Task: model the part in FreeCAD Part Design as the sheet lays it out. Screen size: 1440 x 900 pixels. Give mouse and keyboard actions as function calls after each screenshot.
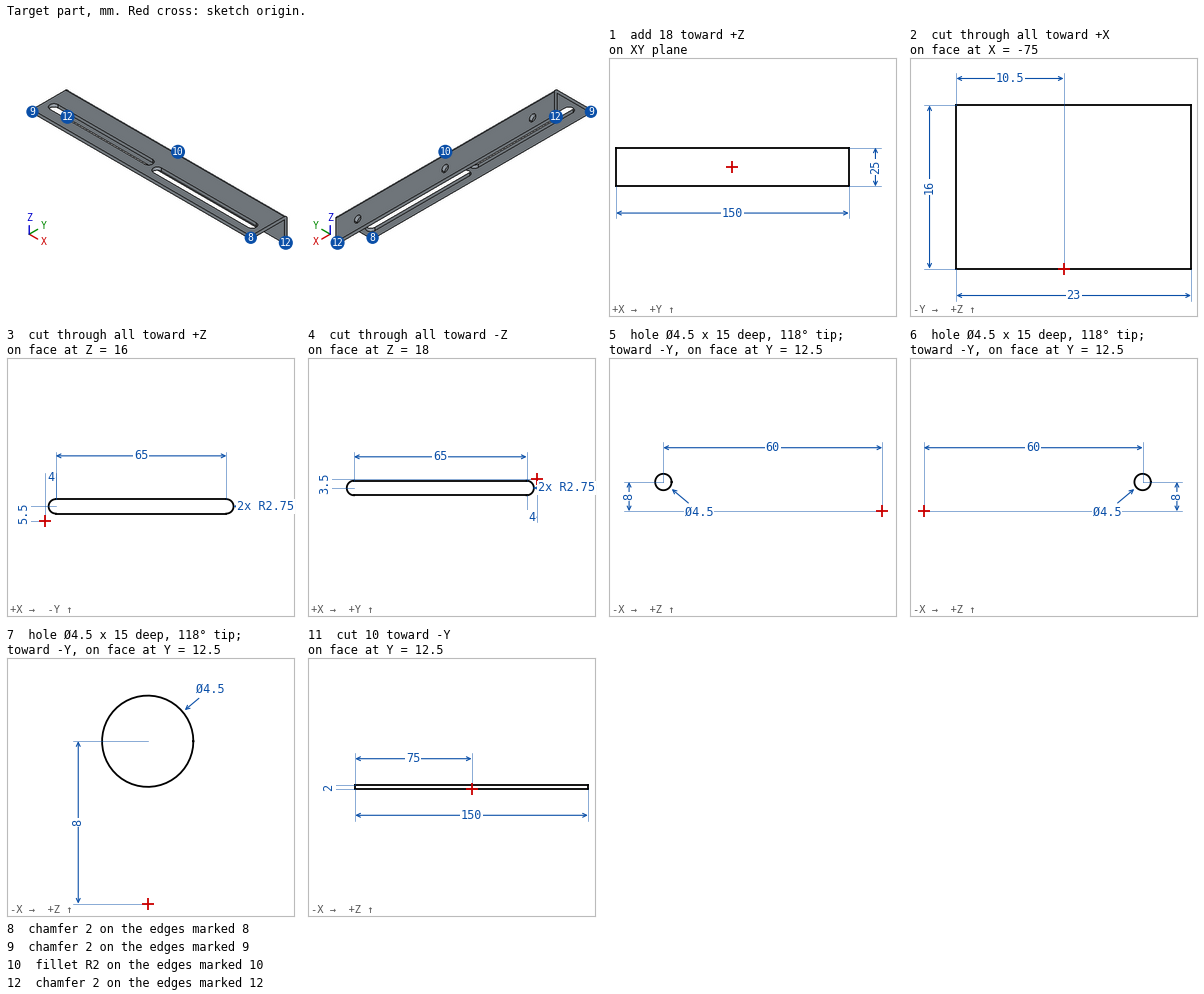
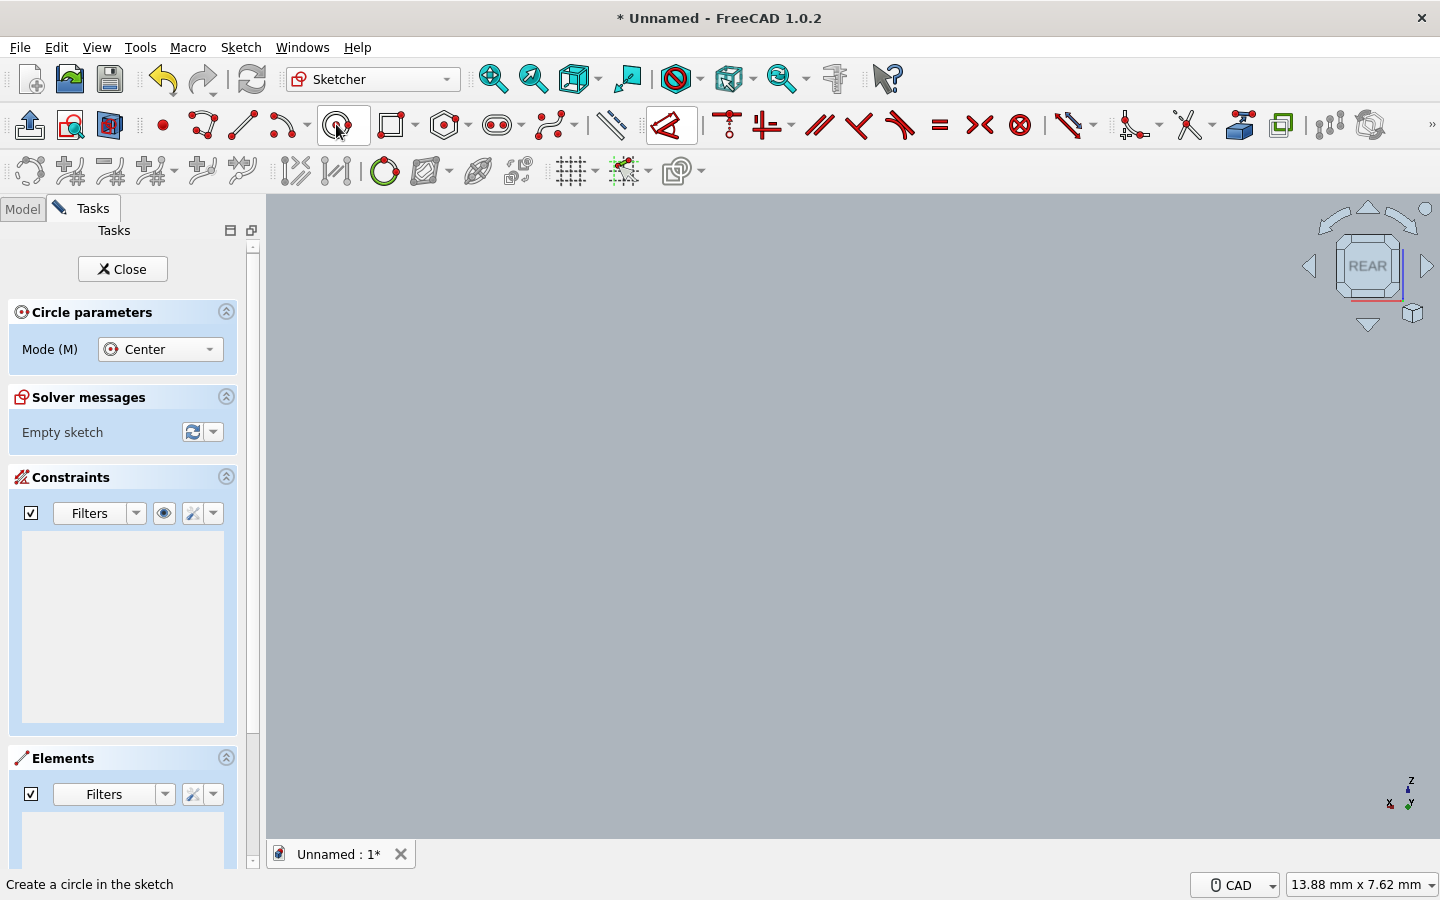
click(776, 506)
move(910, 371)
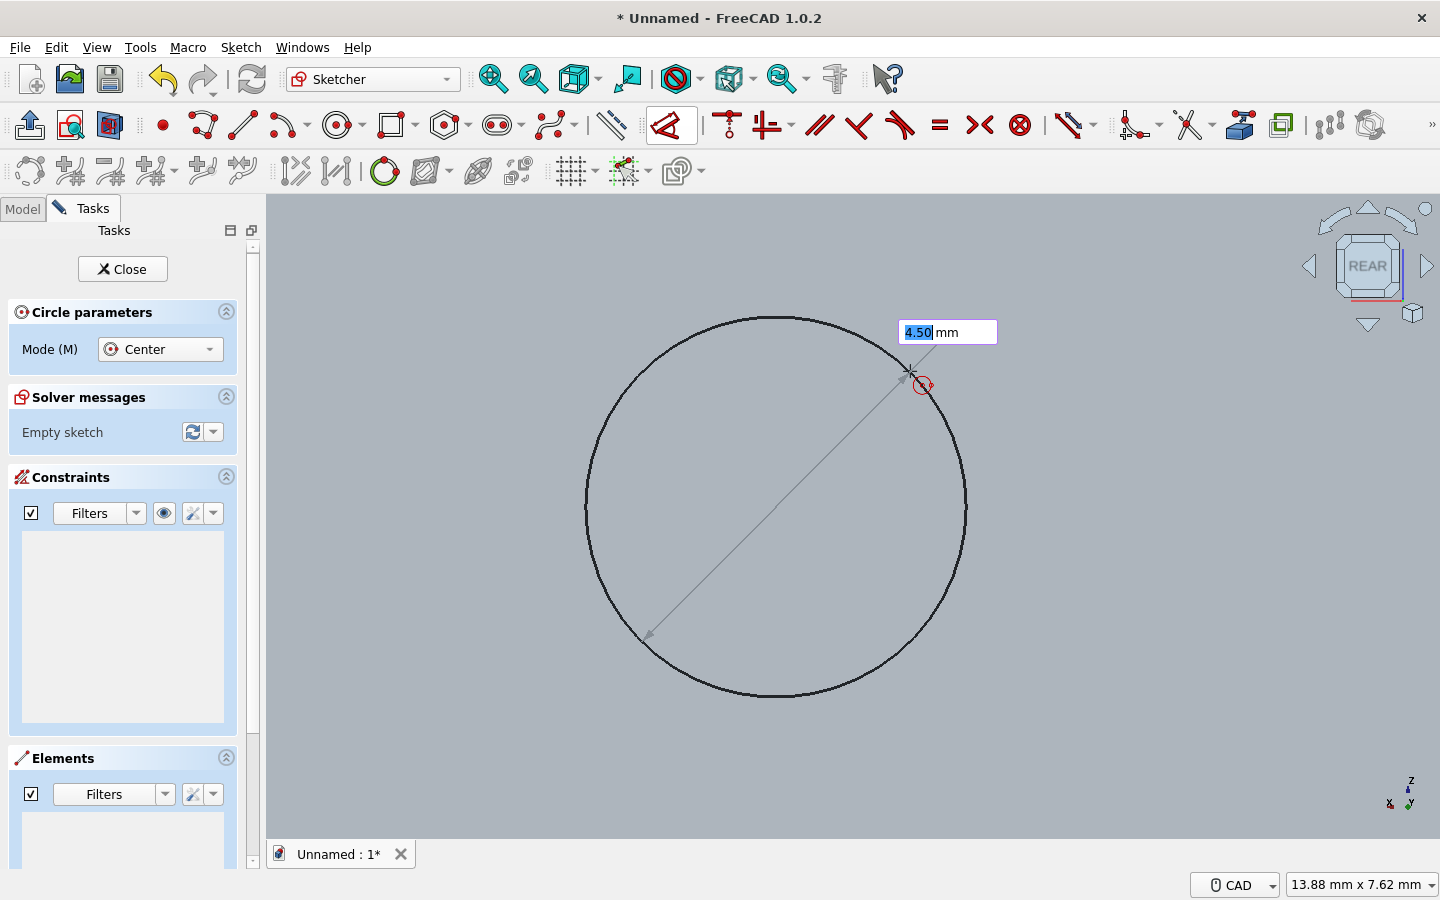
text(4.5)
key(Return)
key(Escape)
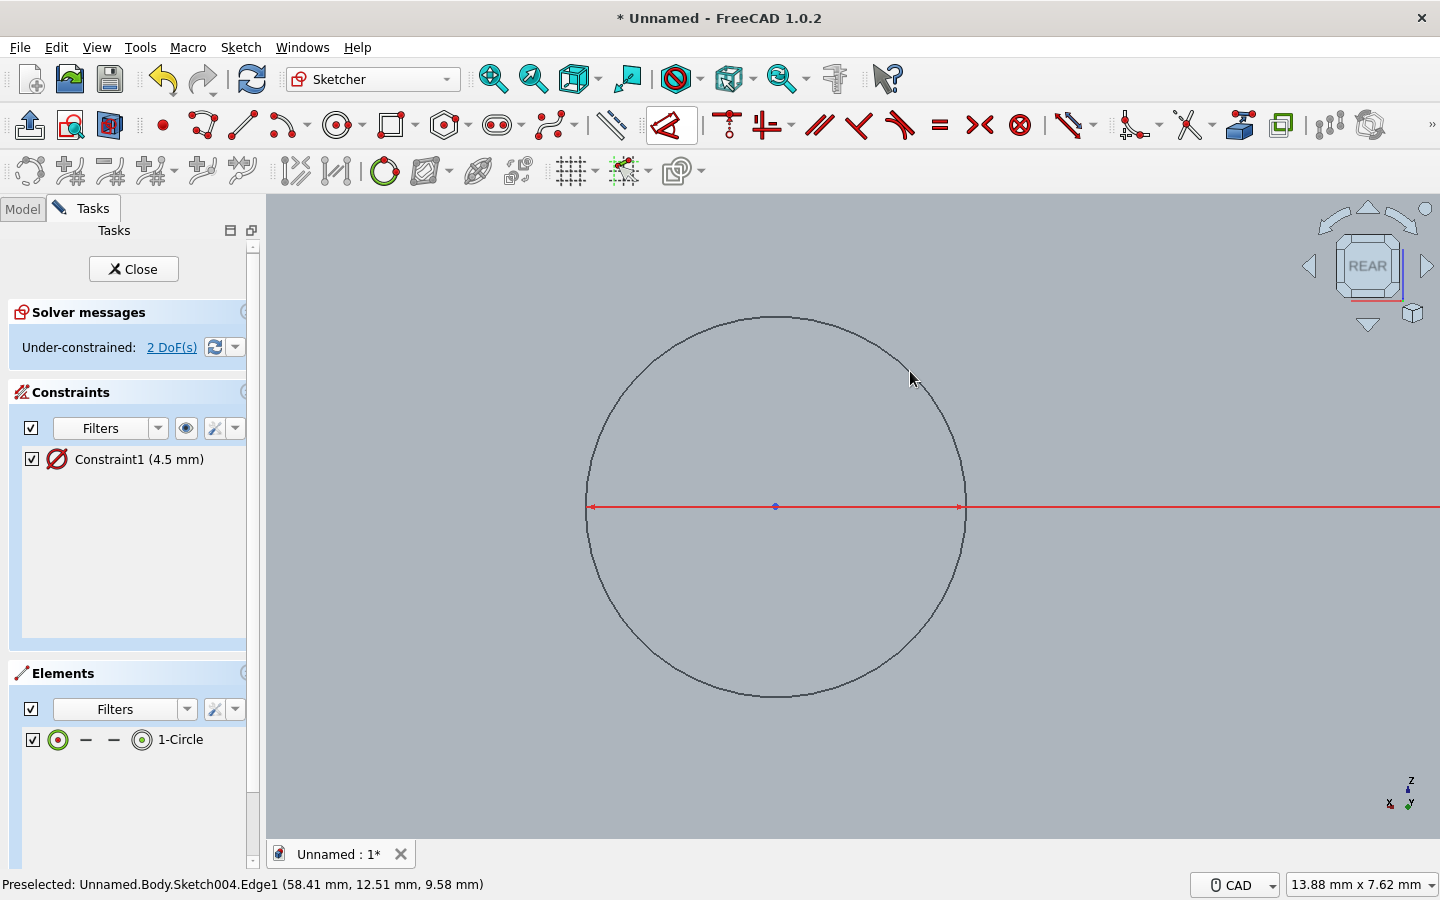
click(776, 507)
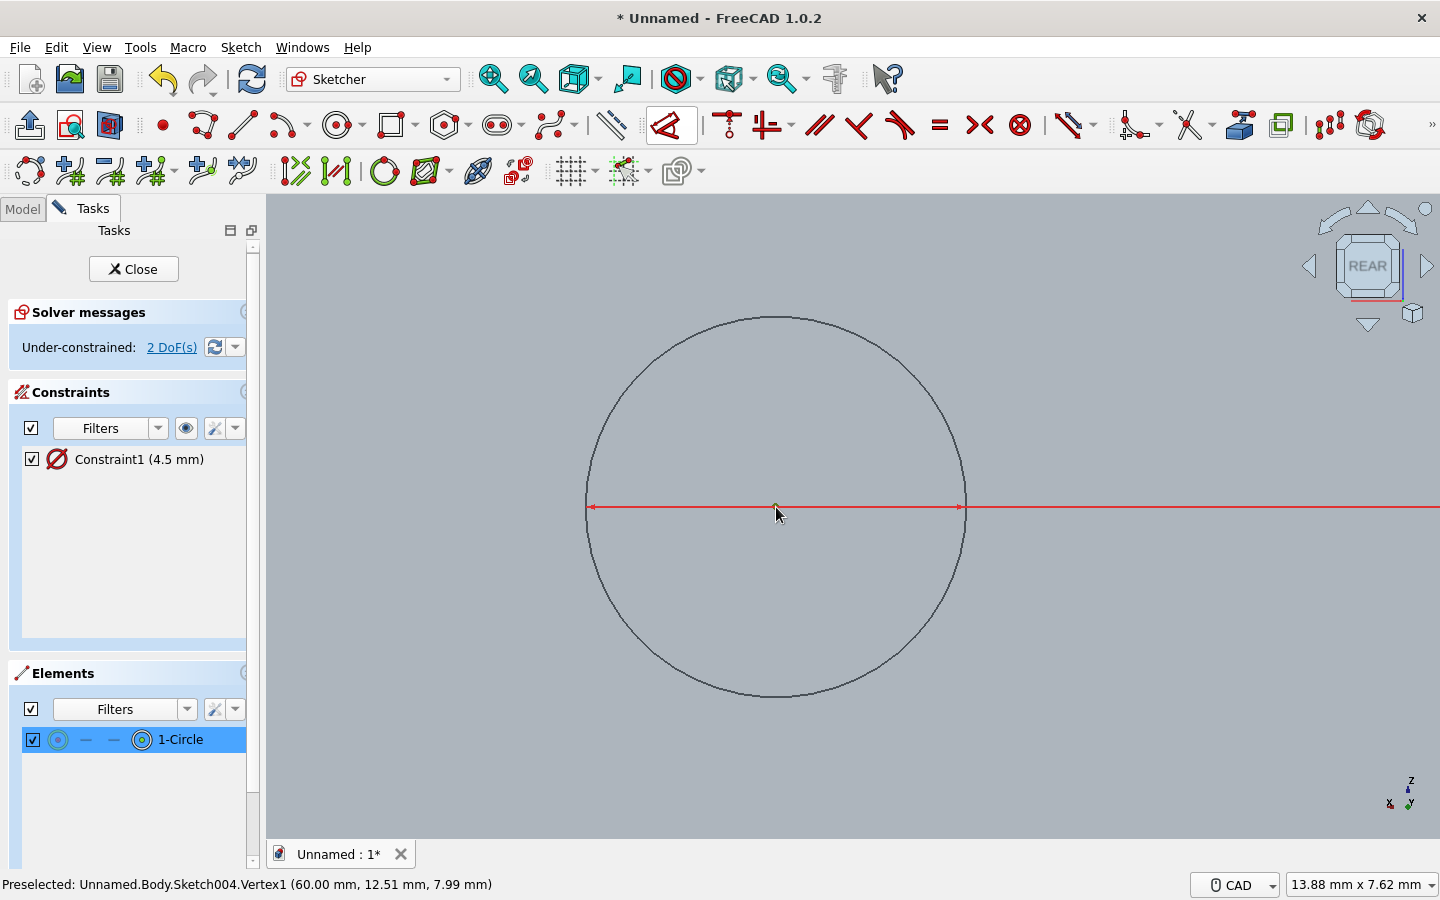
key(i)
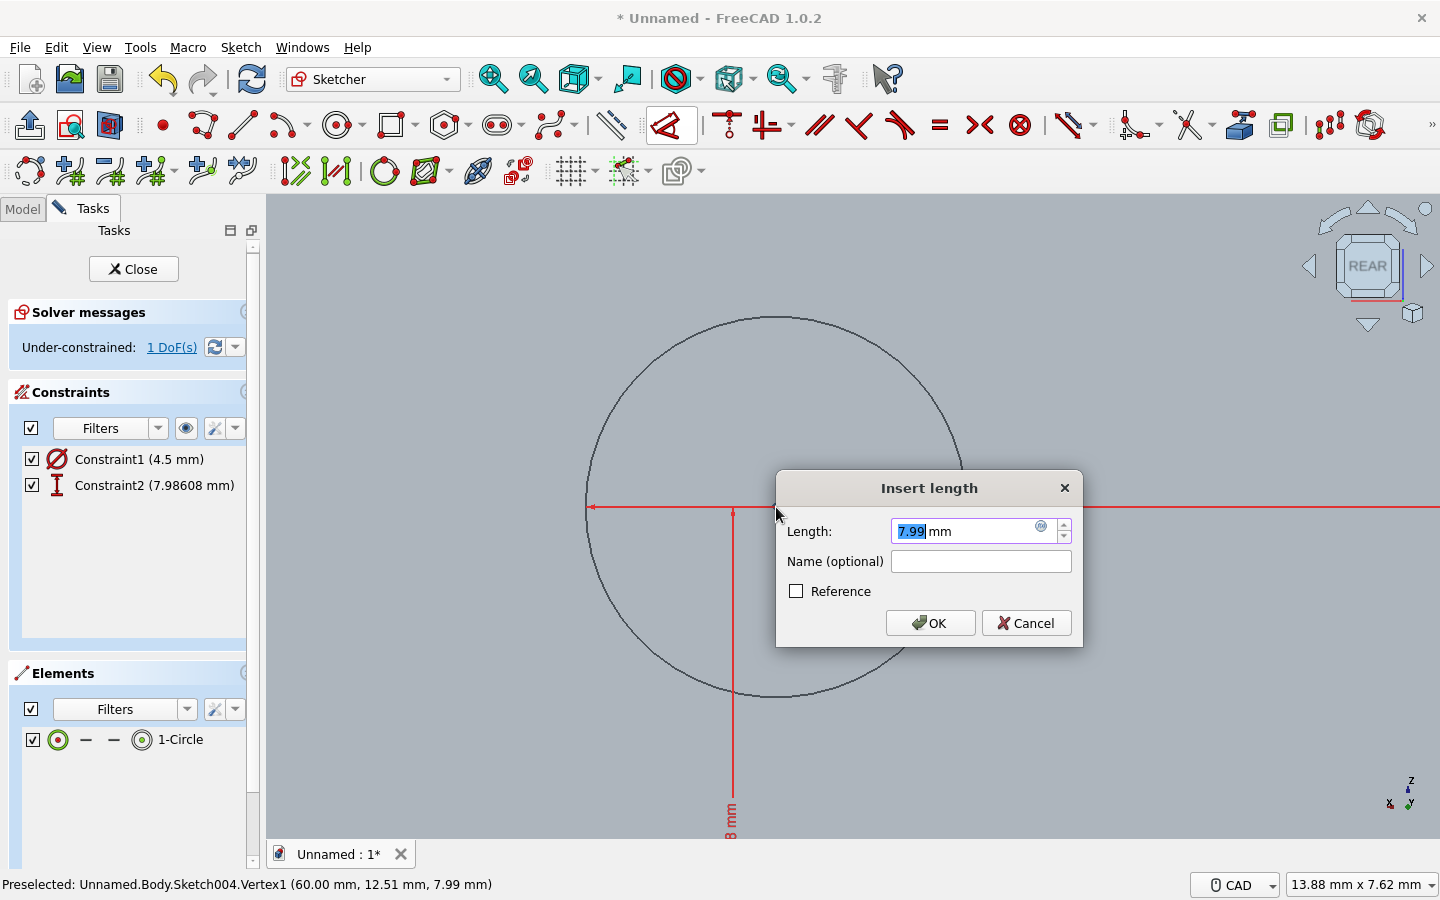
text(8)
key(Return)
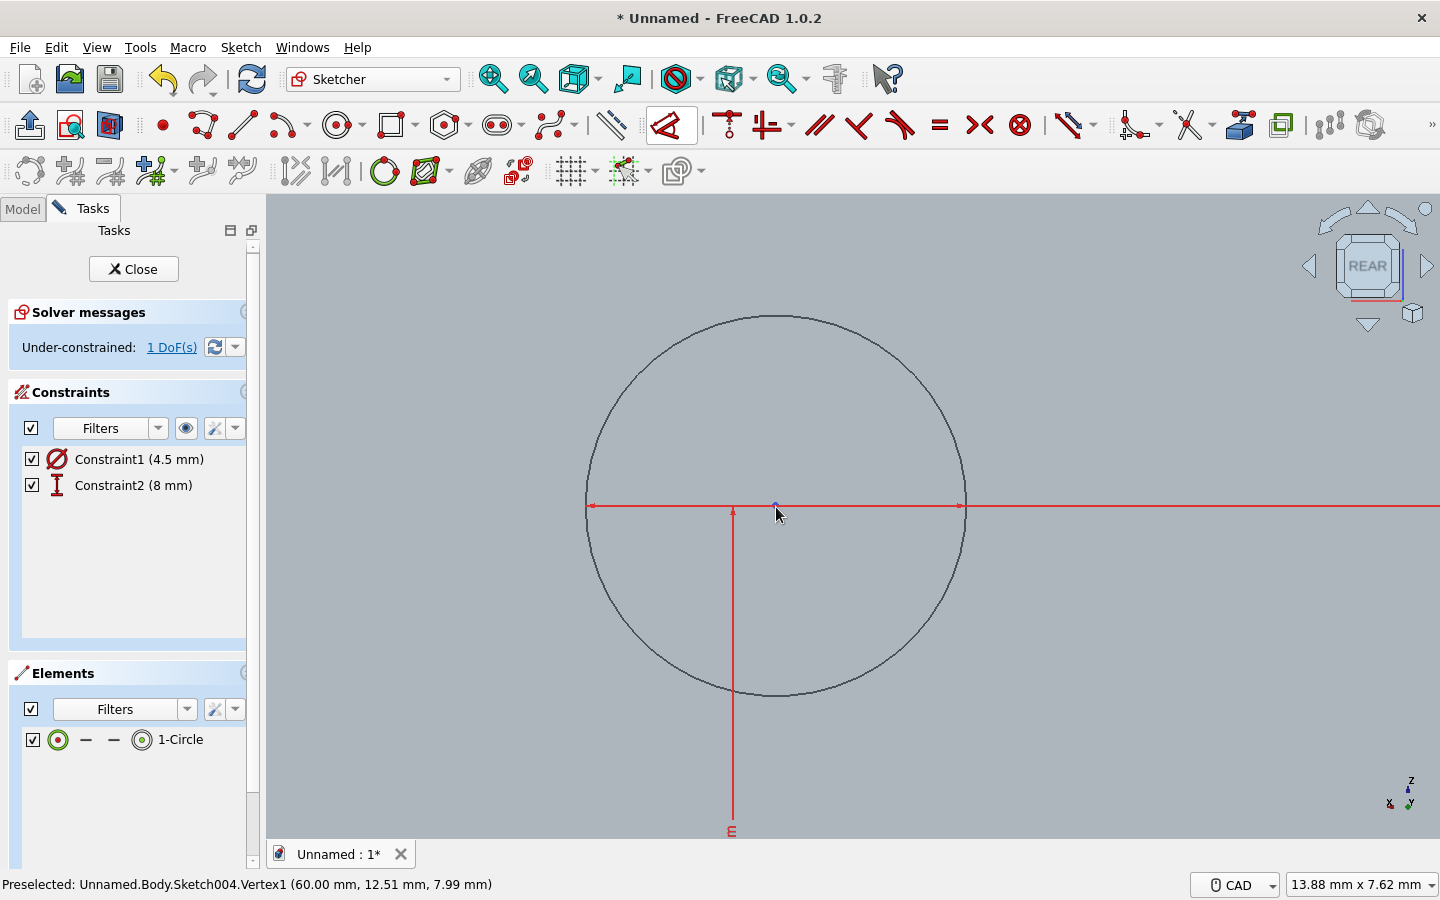
click(776, 506)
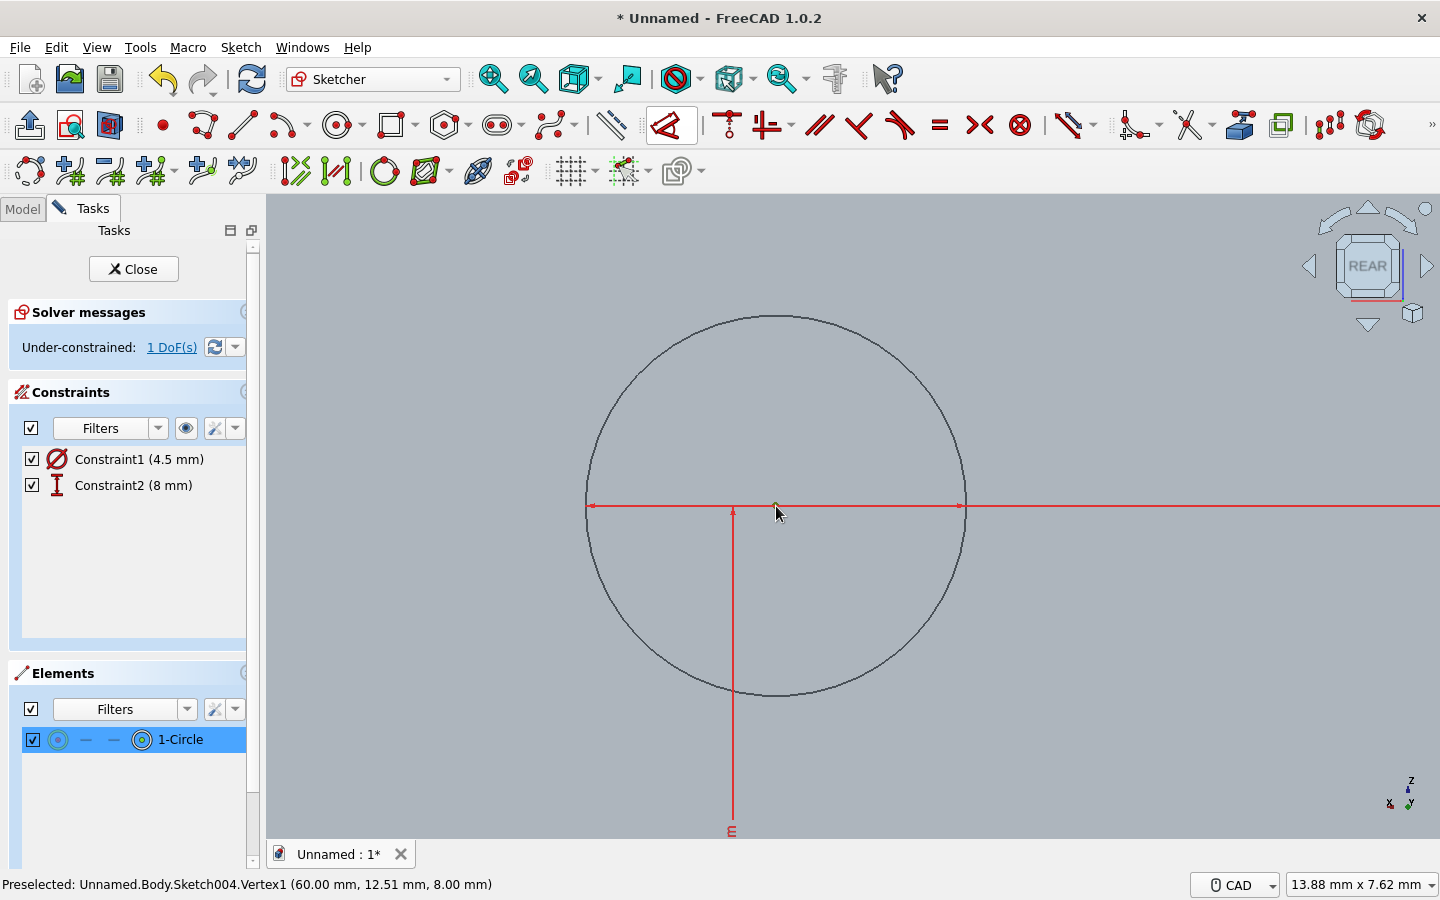
click(692, 126)